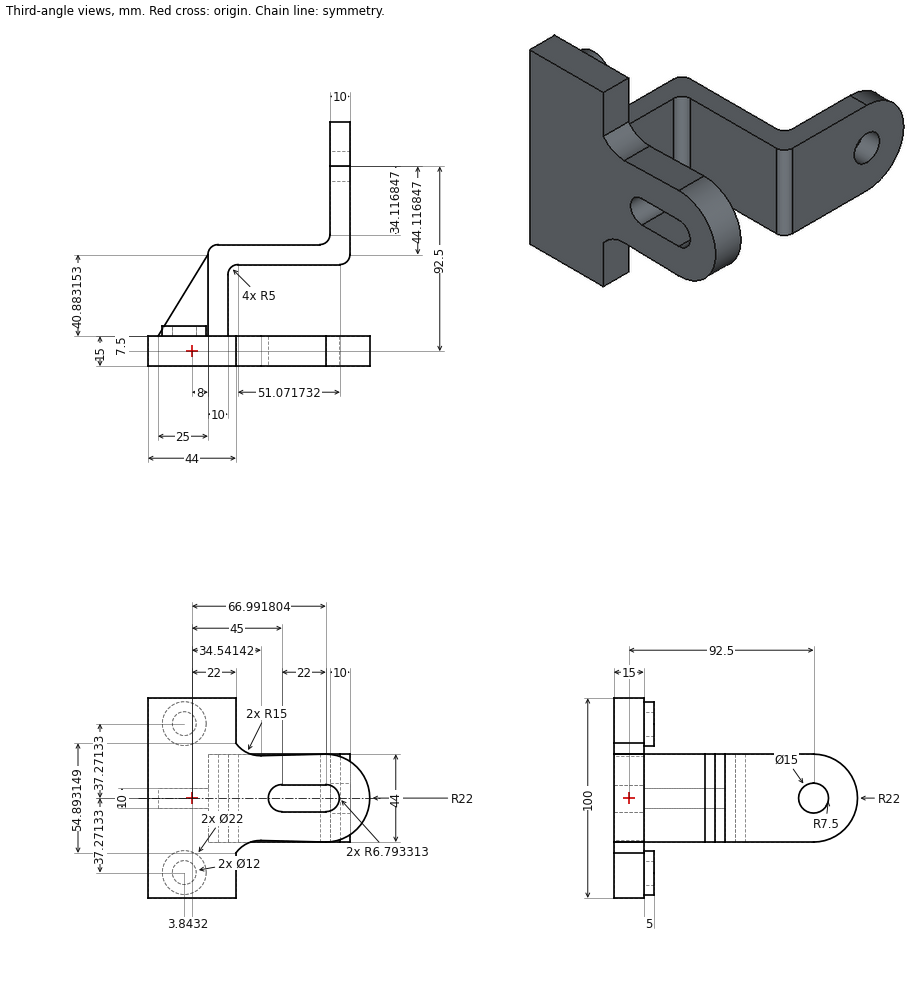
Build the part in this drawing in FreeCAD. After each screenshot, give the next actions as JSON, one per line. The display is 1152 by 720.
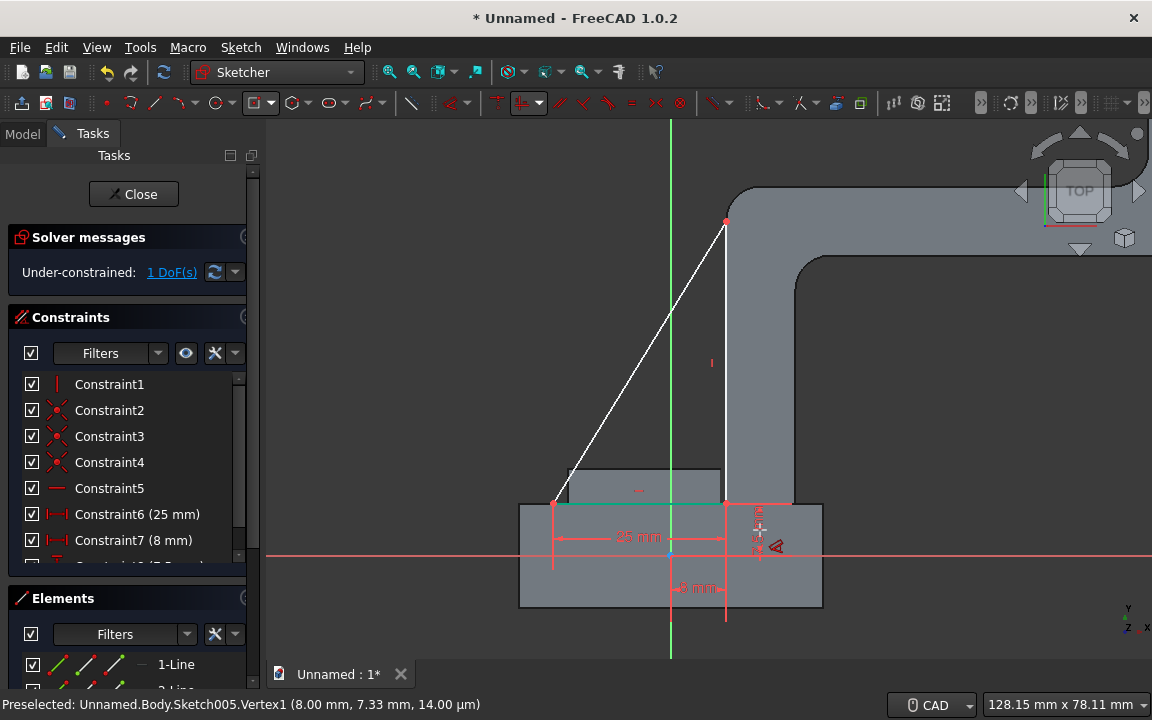
{"action": "left_click", "coordinate": [726, 419]}
{"action": "left_click", "coordinate": [760, 363]}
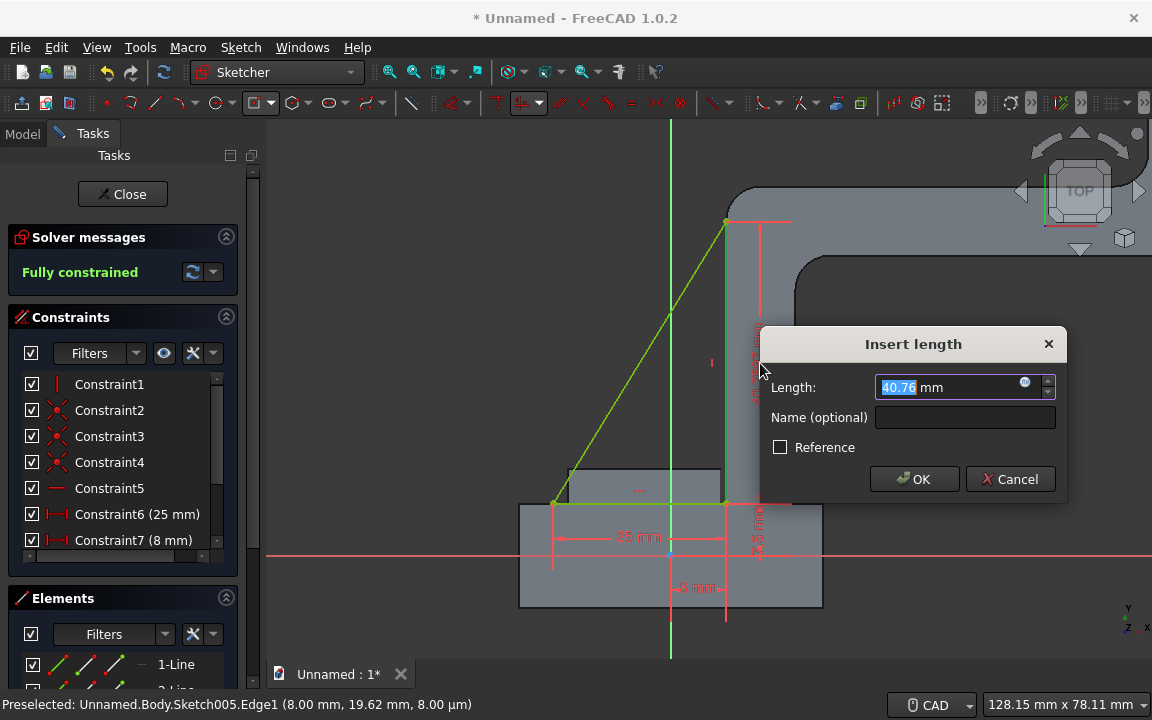
{"action": "type", "text": "40.883153"}
{"action": "key", "text": "Return"}
{"action": "key", "text": "Escape"}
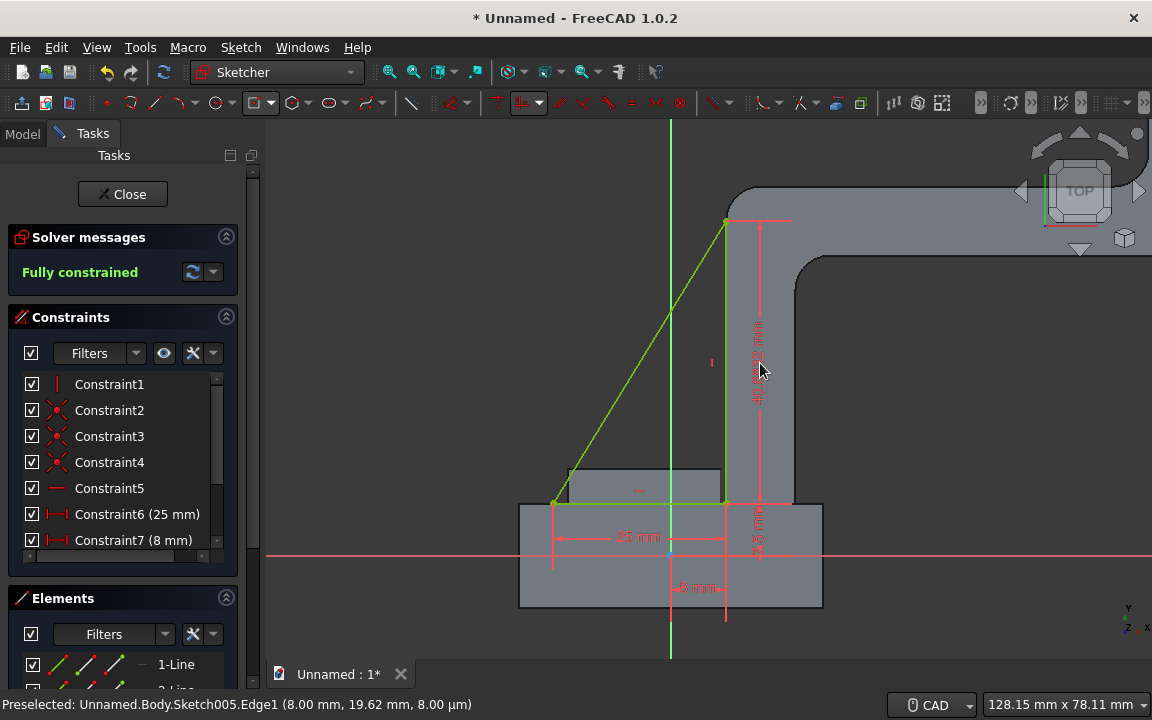
{"action": "left_click", "coordinate": [123, 194]}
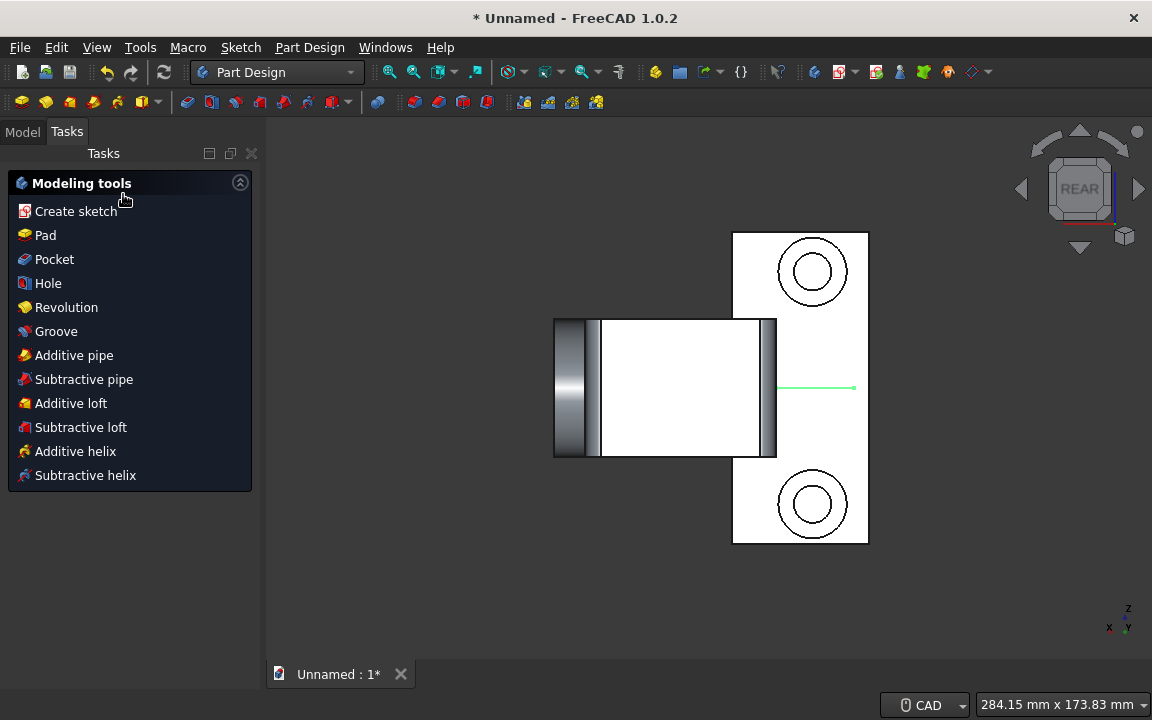
{"action": "left_click", "coordinate": [22, 102]}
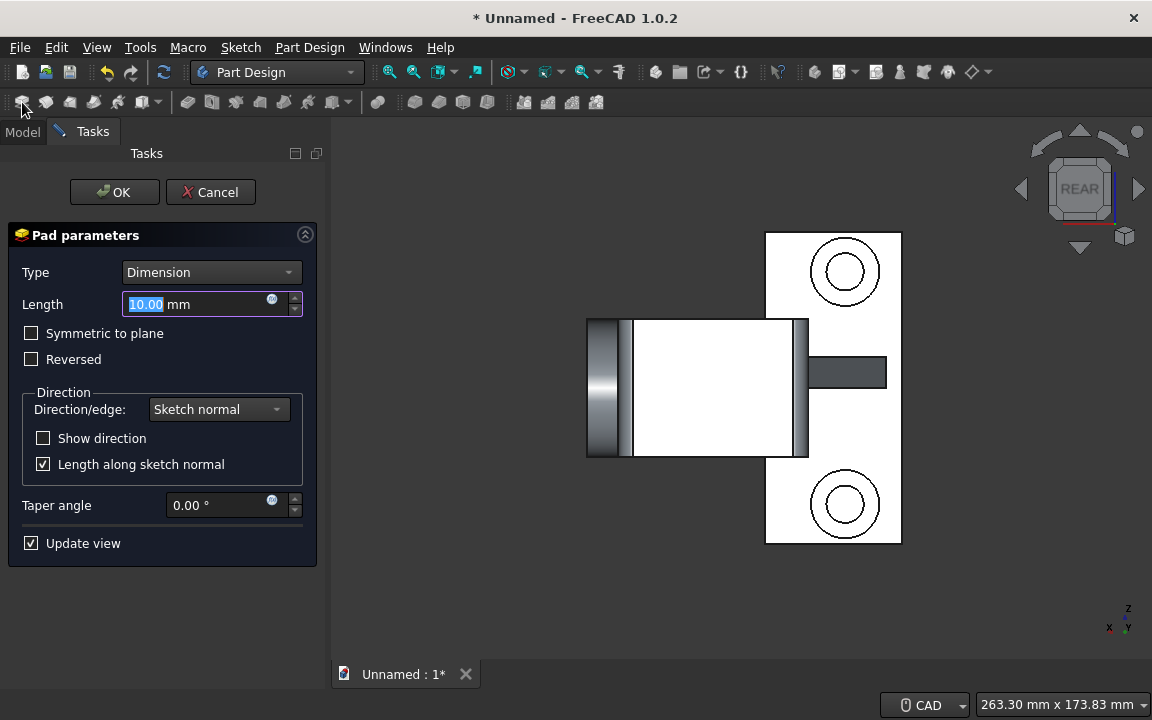
{"action": "type", "text": "10"}
{"action": "key", "text": "Tab"}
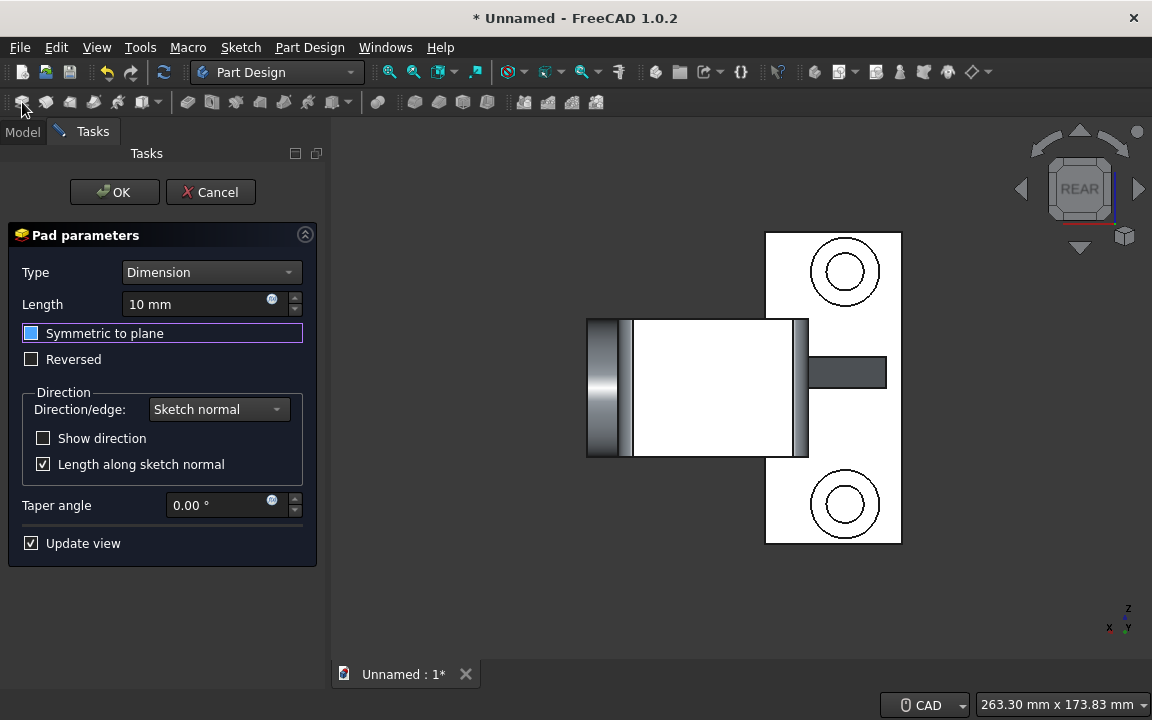
{"action": "left_click", "coordinate": [30, 333]}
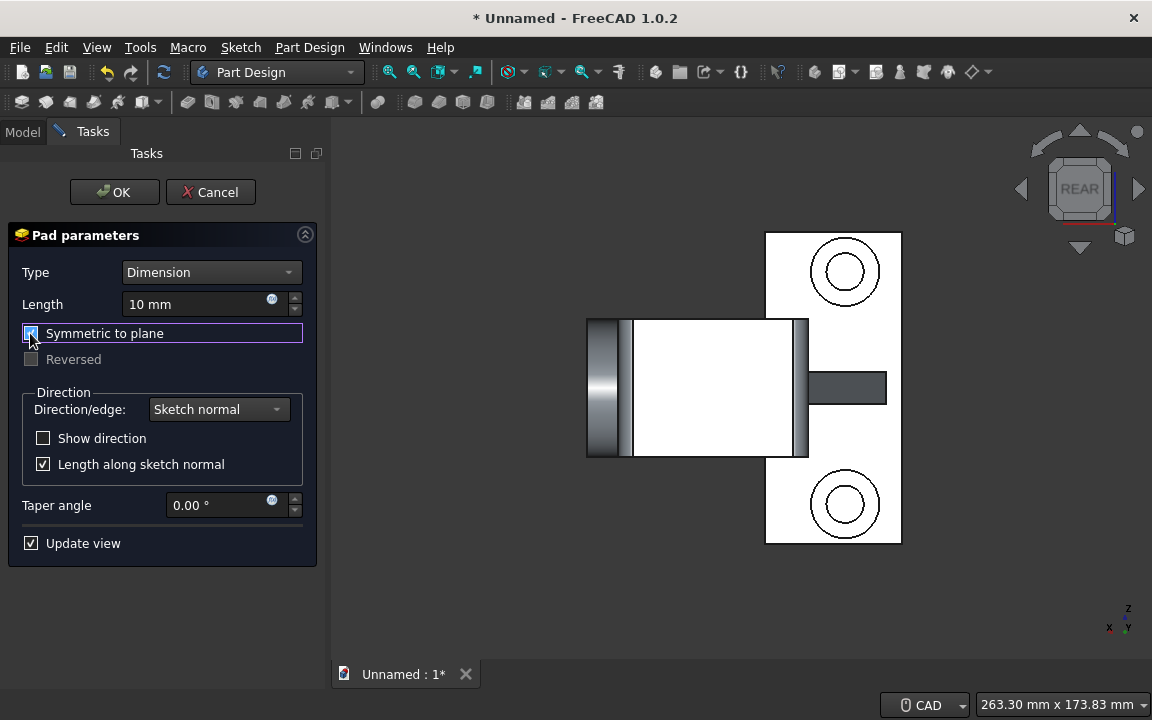
{"action": "left_click", "coordinate": [115, 192]}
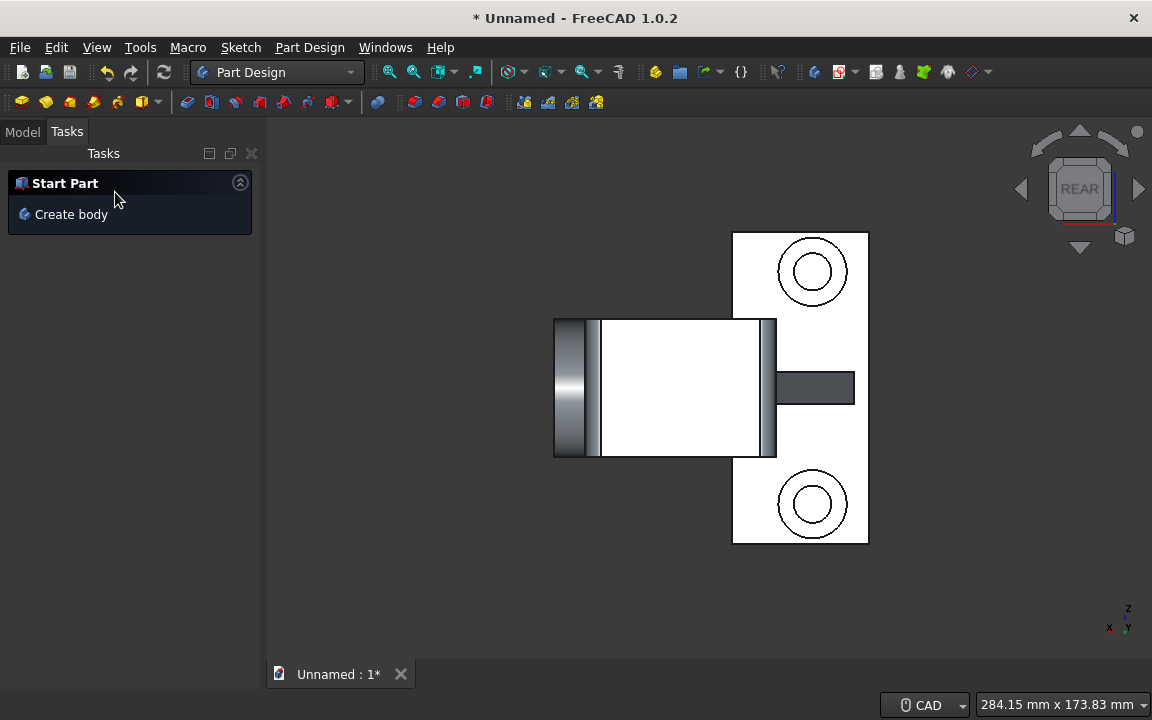
{"action": "key", "text": "0"}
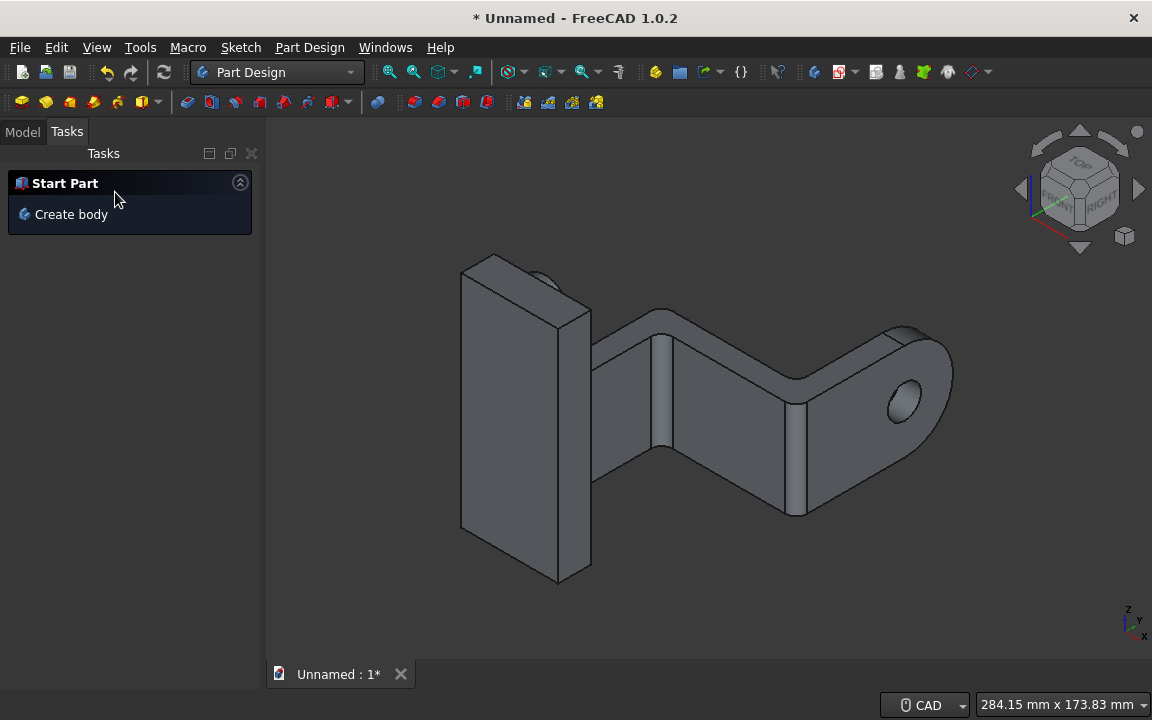
{"action": "left_click", "coordinate": [510, 391]}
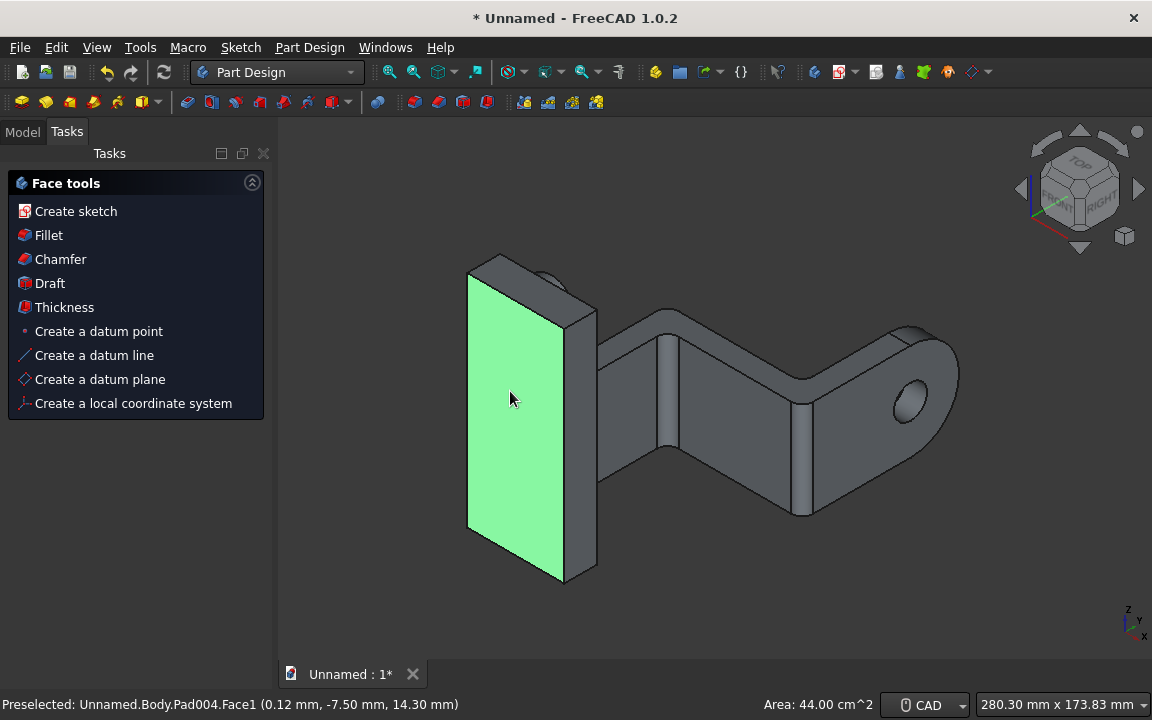
{"action": "left_click", "coordinate": [840, 72]}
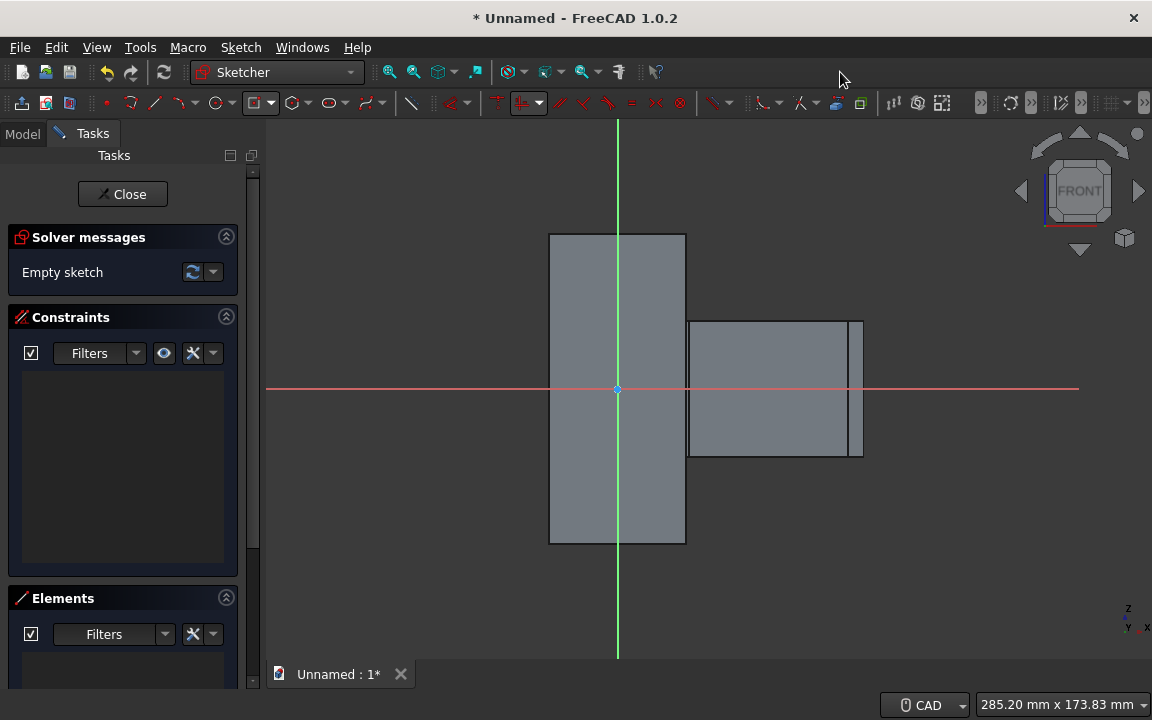
{"action": "scroll", "coordinate": [896, 389], "scroll_direction": "up", "scroll_amount": 3}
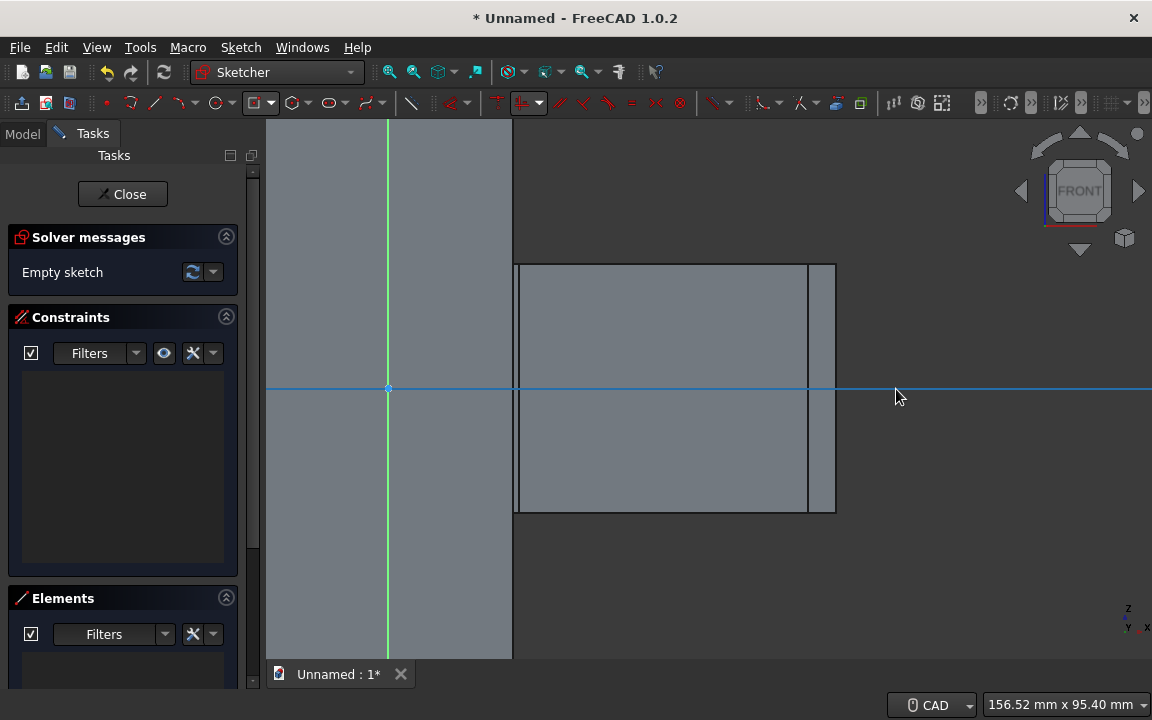
{"action": "left_click", "coordinate": [156, 104]}